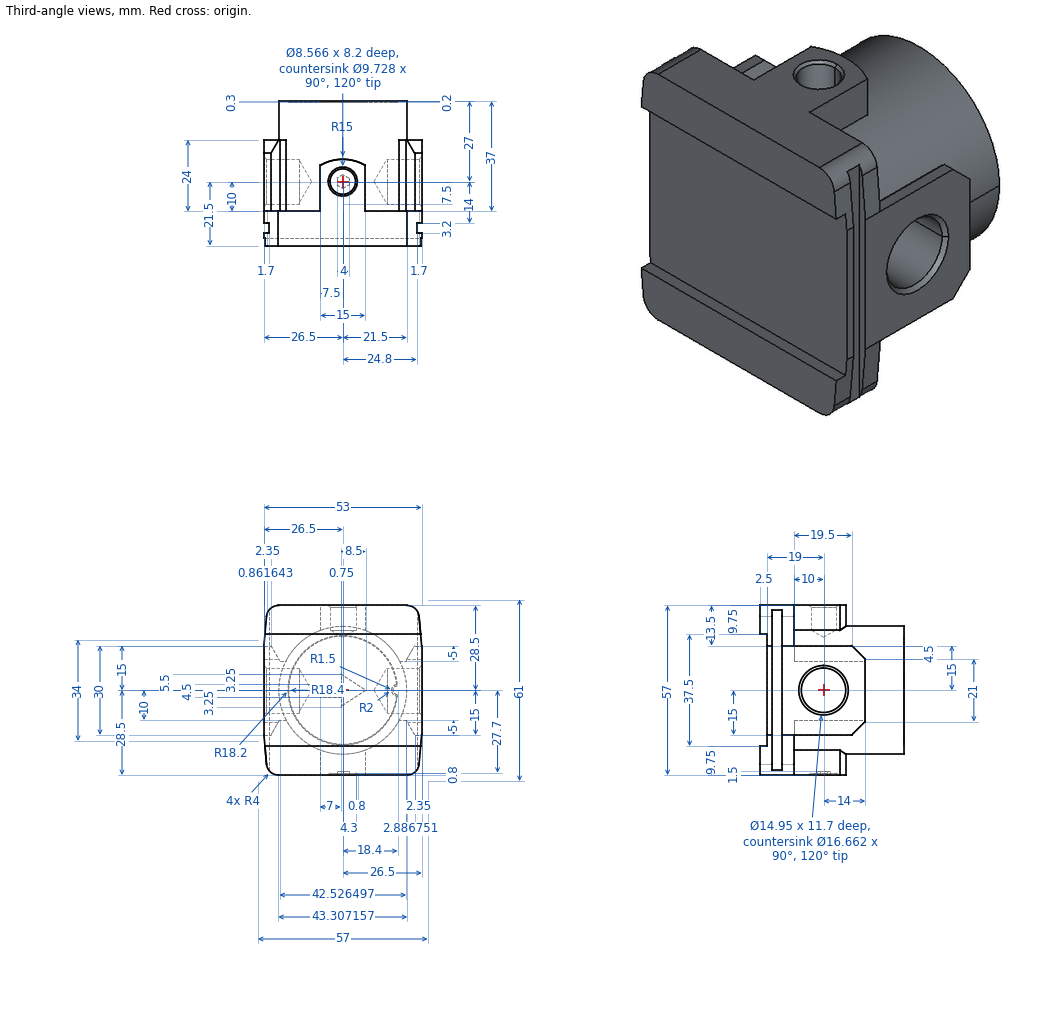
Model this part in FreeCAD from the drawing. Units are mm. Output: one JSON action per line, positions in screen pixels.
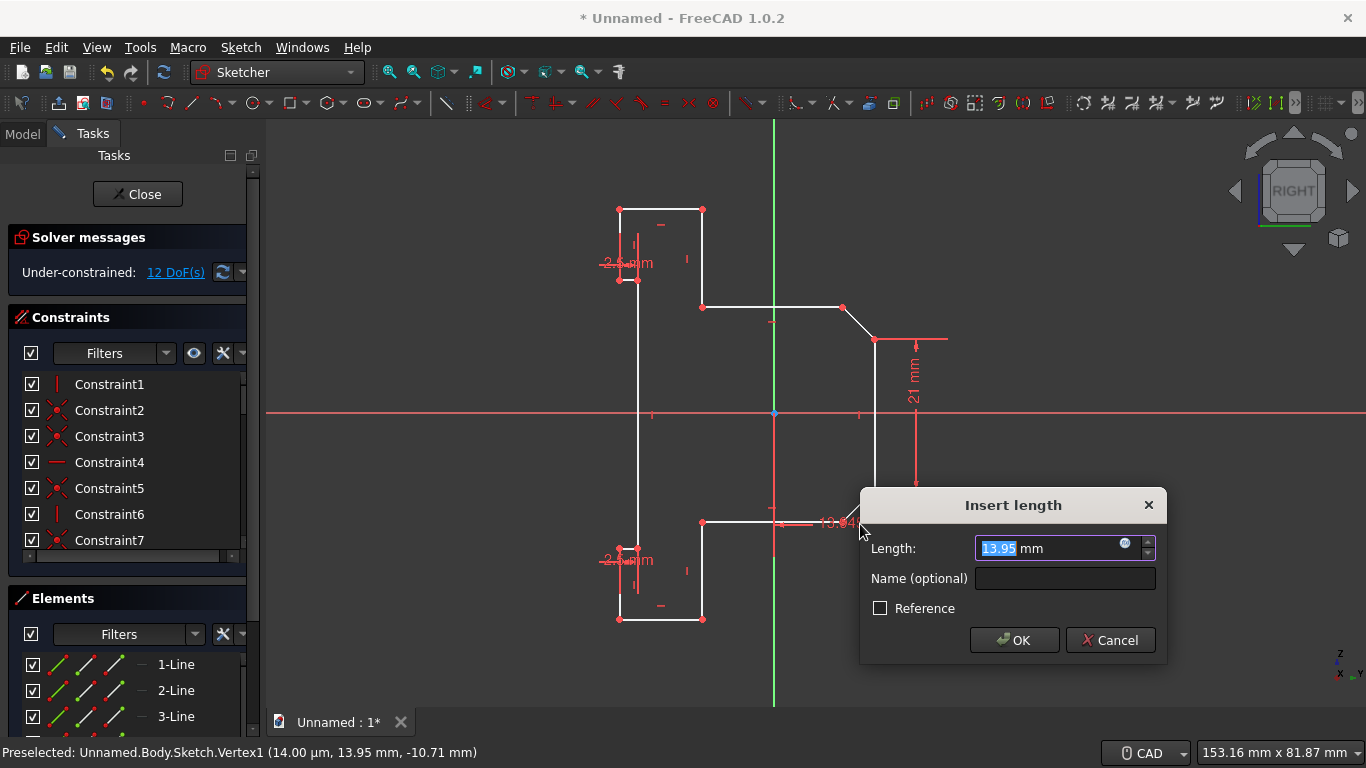
{"action": "type", "text": "14"}
{"action": "key", "text": "Return"}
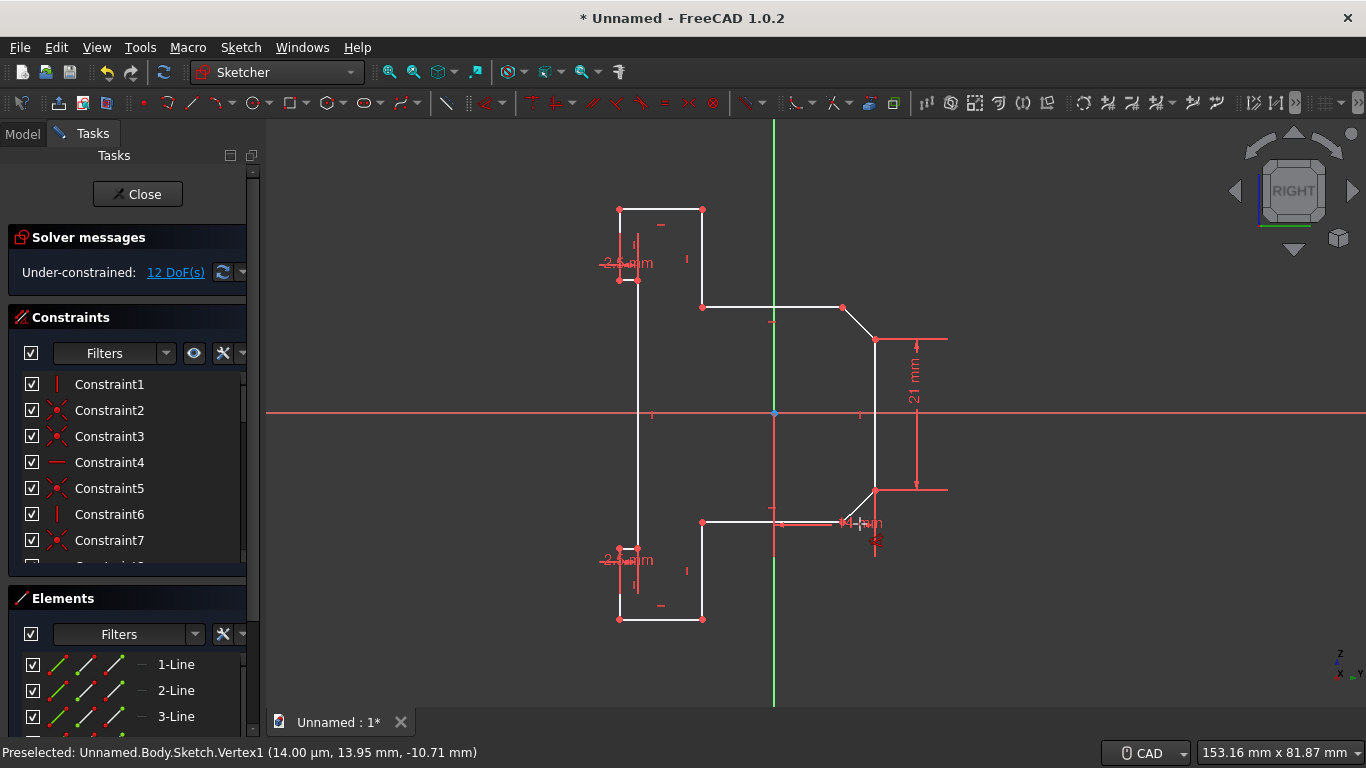
{"action": "left_click", "coordinate": [843, 307]}
{"action": "left_click", "coordinate": [740, 360]}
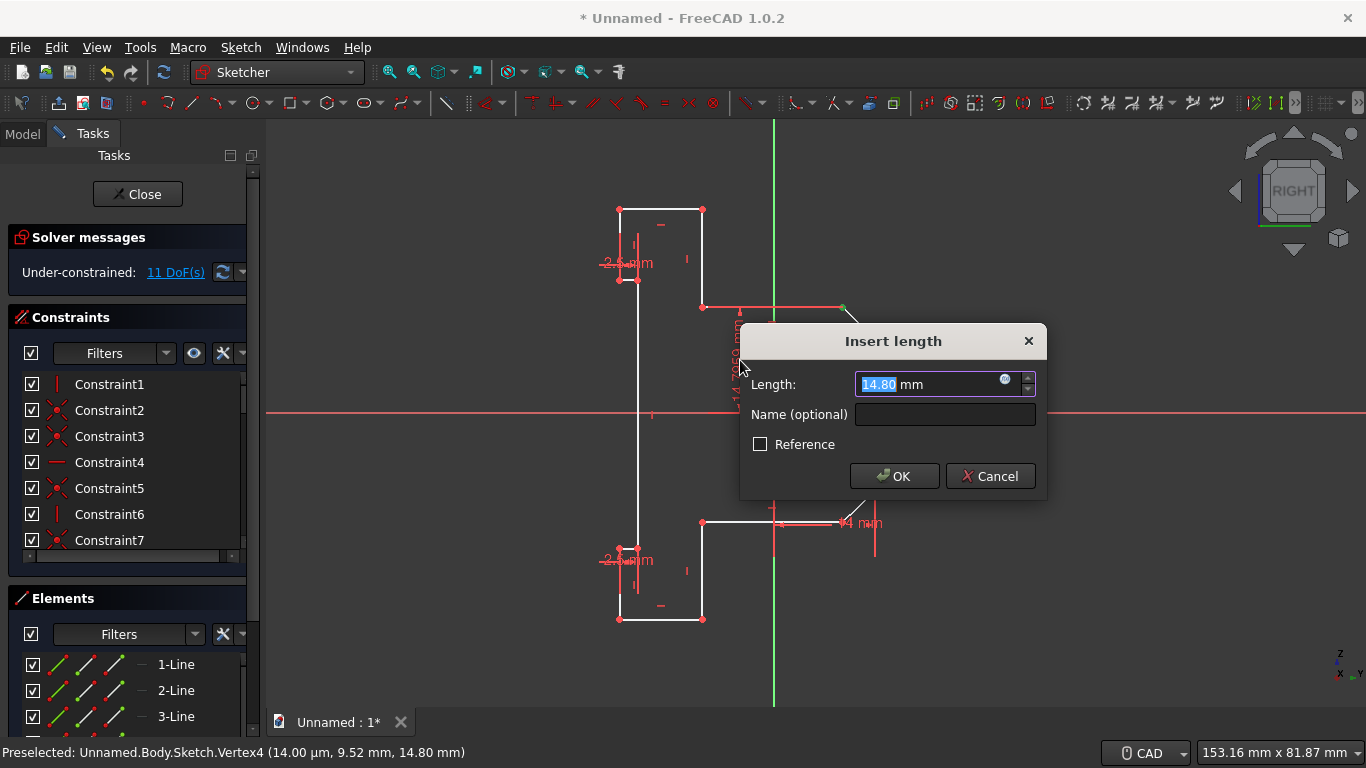
{"action": "type", "text": "15"}
{"action": "key", "text": "Return"}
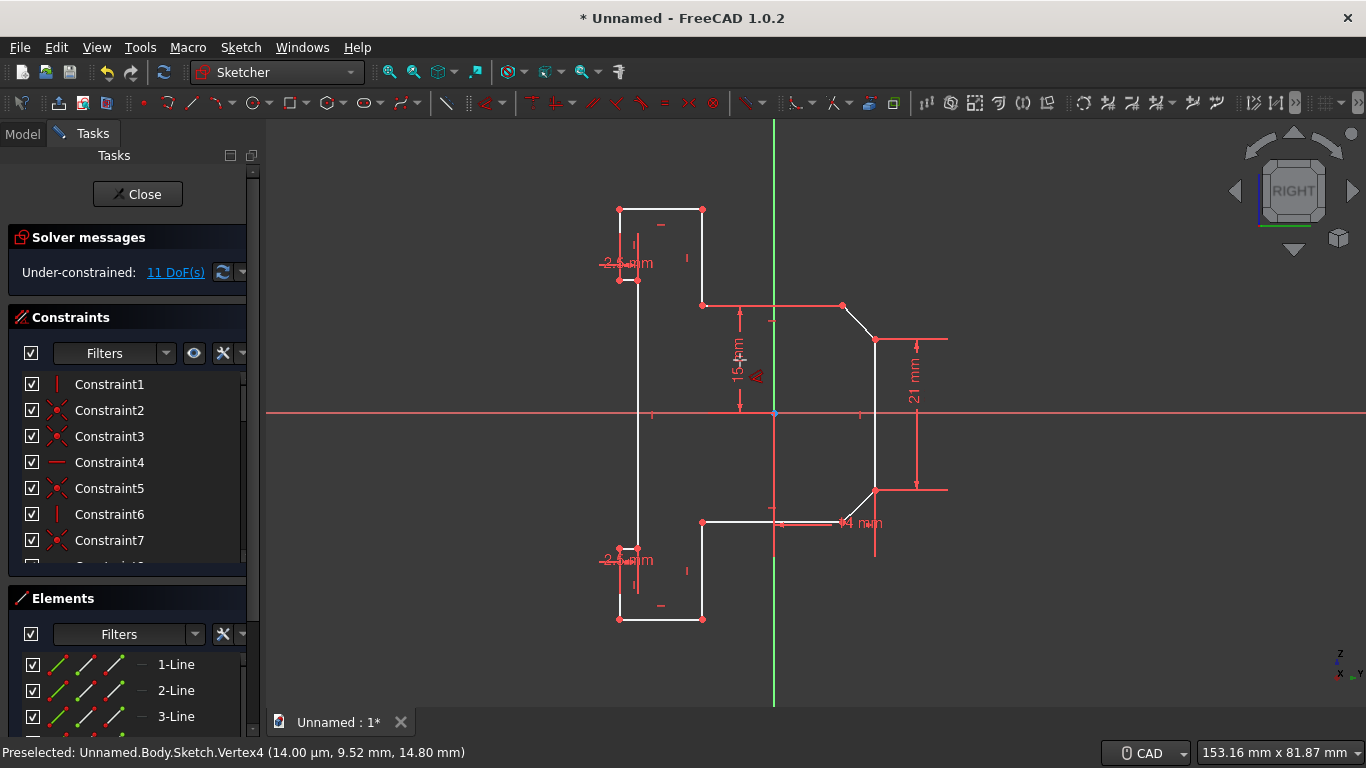
{"action": "left_click", "coordinate": [702, 306]}
{"action": "left_click", "coordinate": [738, 272]}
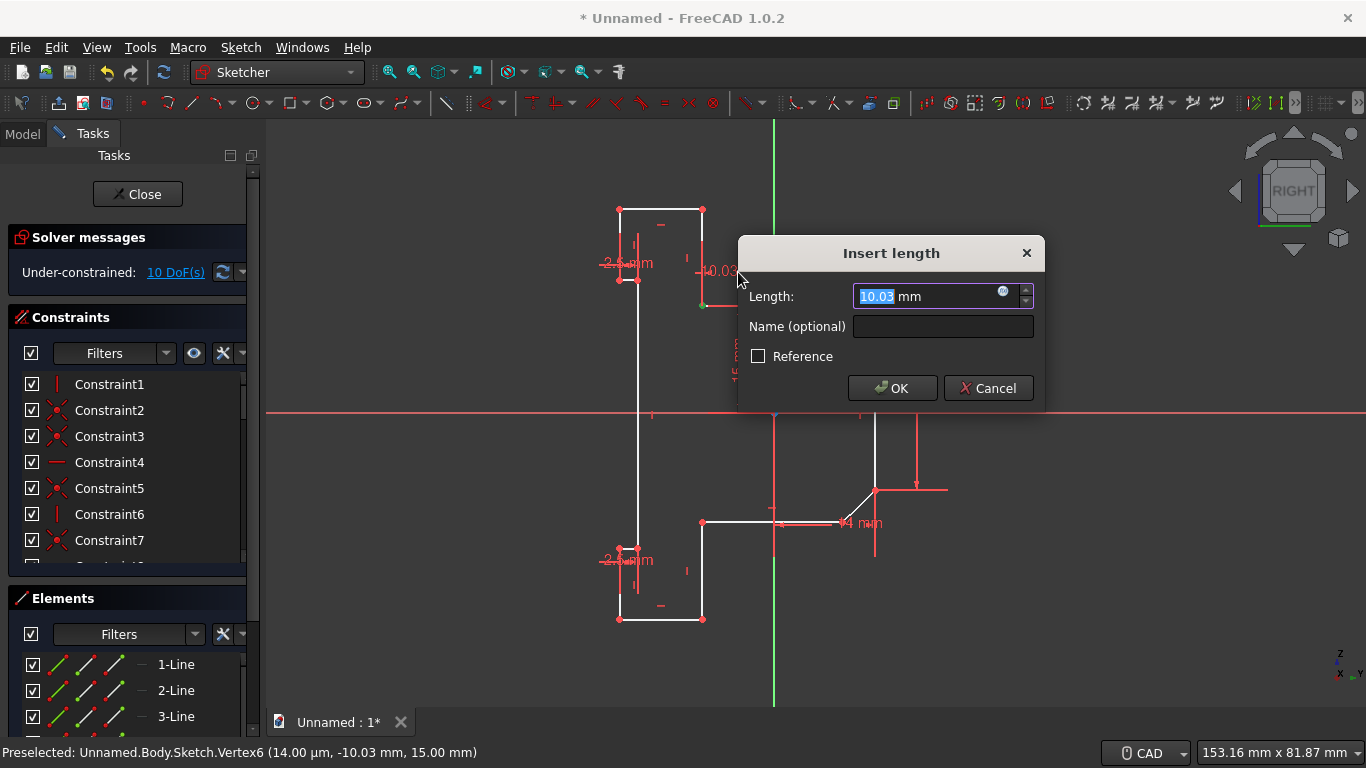
{"action": "type", "text": "10"}
{"action": "key", "text": "Return"}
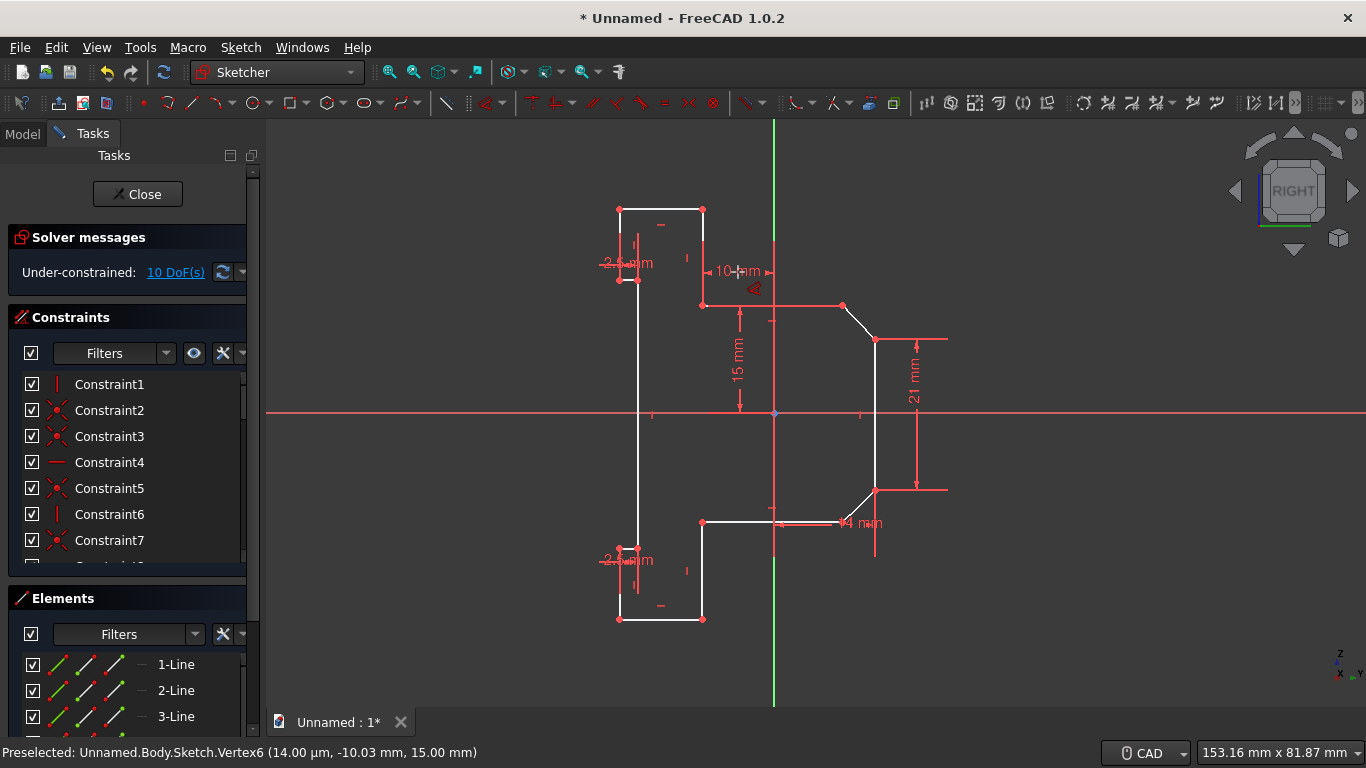
{"action": "left_click", "coordinate": [638, 280]}
{"action": "left_click", "coordinate": [738, 246]}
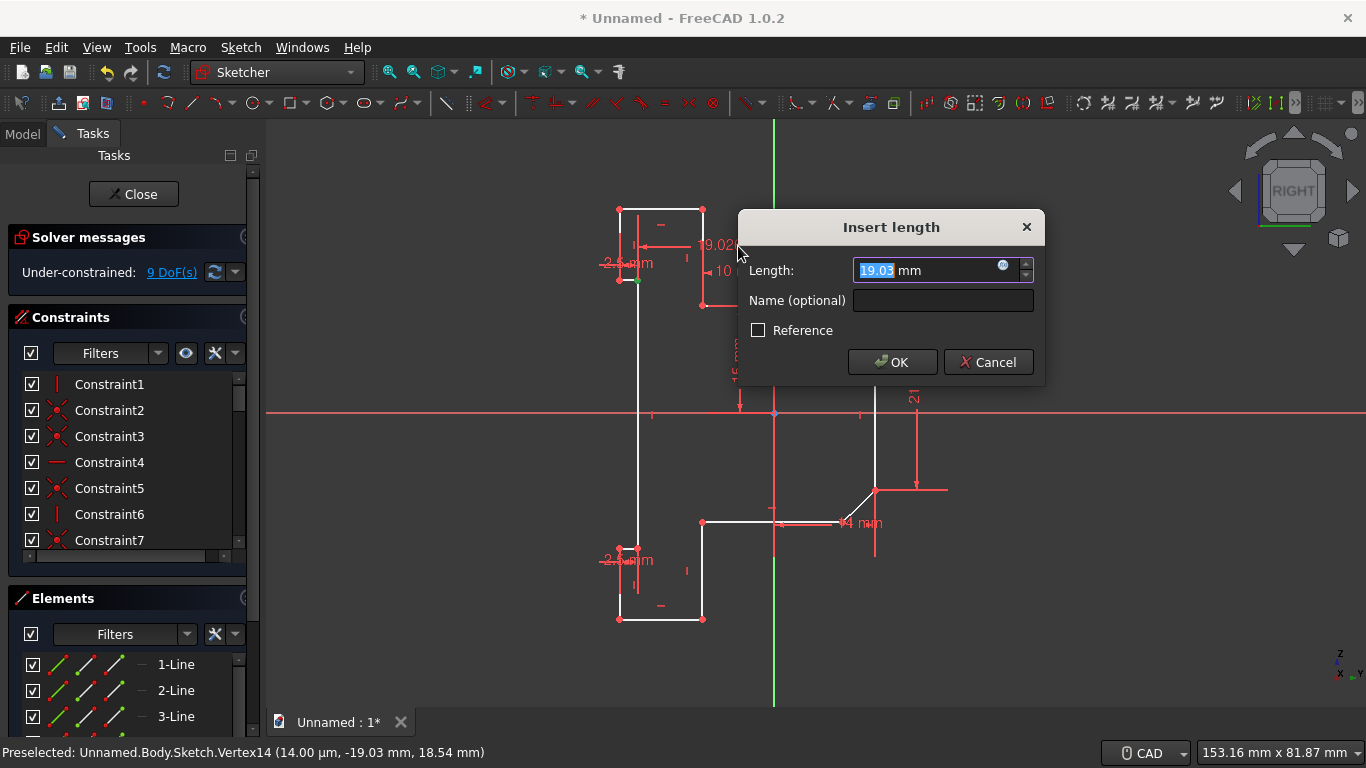
{"action": "type", "text": "19"}
{"action": "key", "text": "Return"}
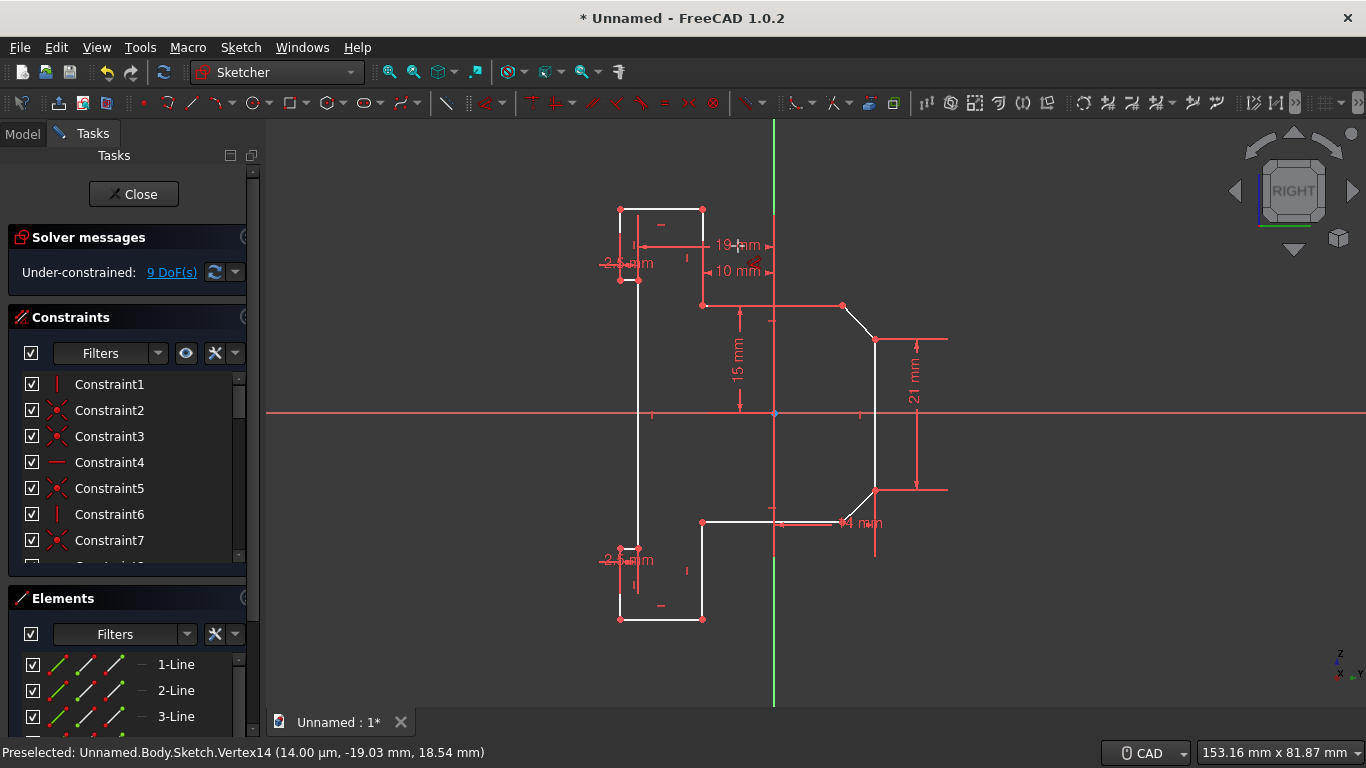
{"action": "left_click", "coordinate": [702, 620]}
{"action": "left_click", "coordinate": [738, 654]}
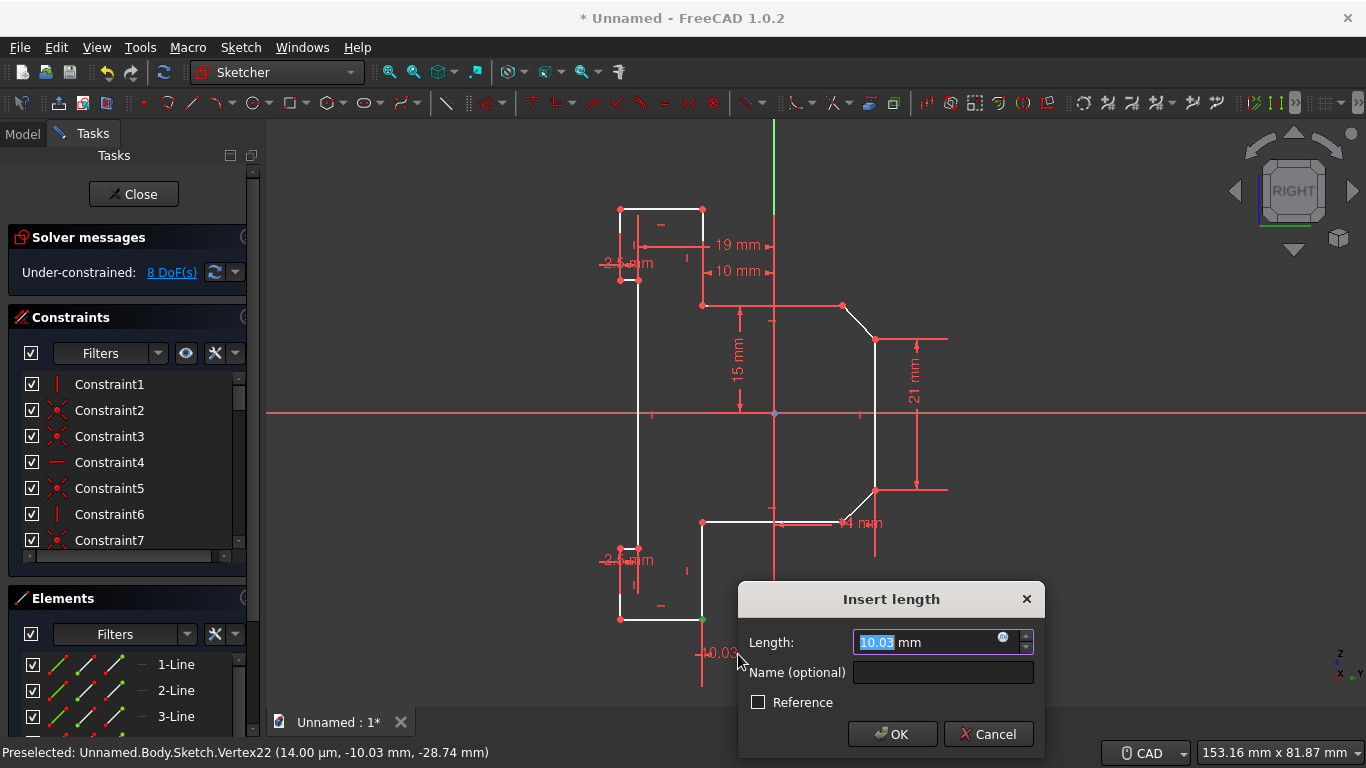
{"action": "type", "text": "10"}
{"action": "key", "text": "Return"}